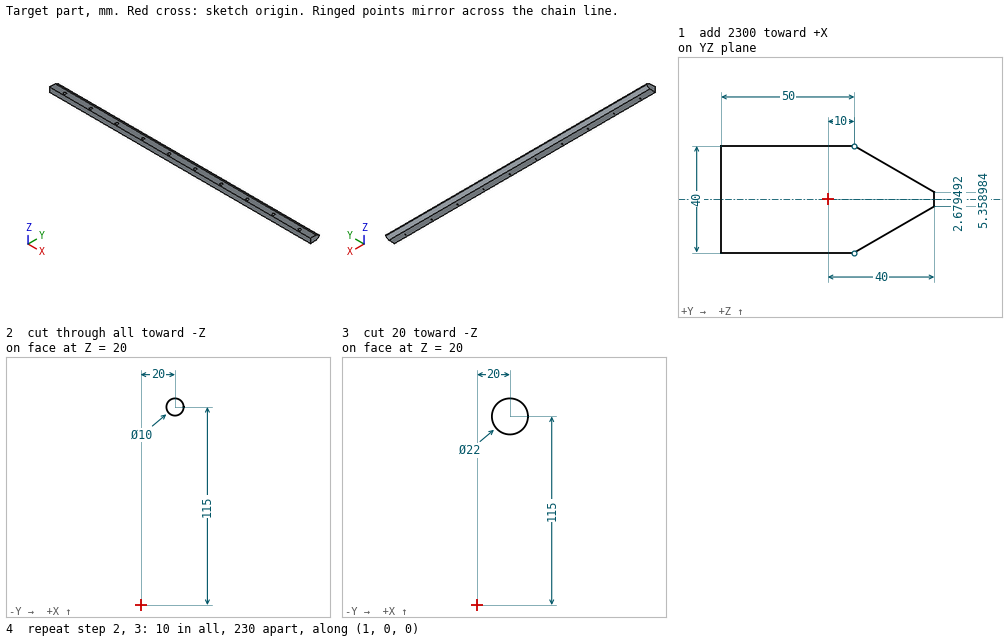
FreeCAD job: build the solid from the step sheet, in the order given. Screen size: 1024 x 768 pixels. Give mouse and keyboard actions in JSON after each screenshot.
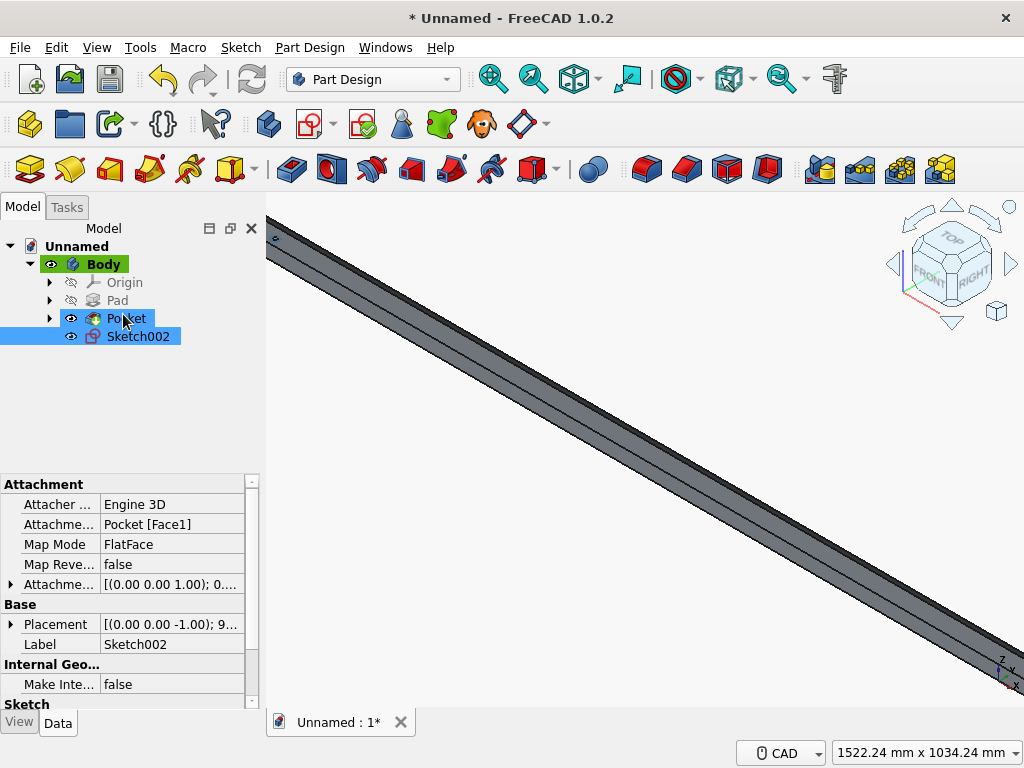
{"action": "left_click", "coordinate": [292, 170]}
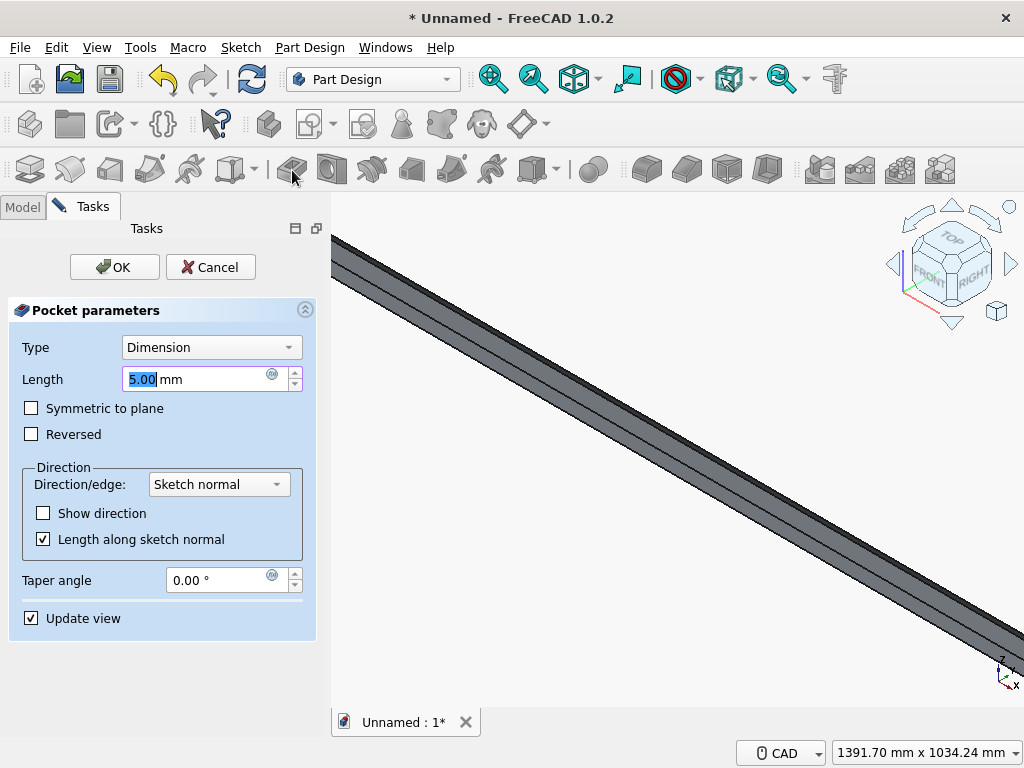
{"action": "type", "text": "20"}
{"action": "key", "text": "Tab"}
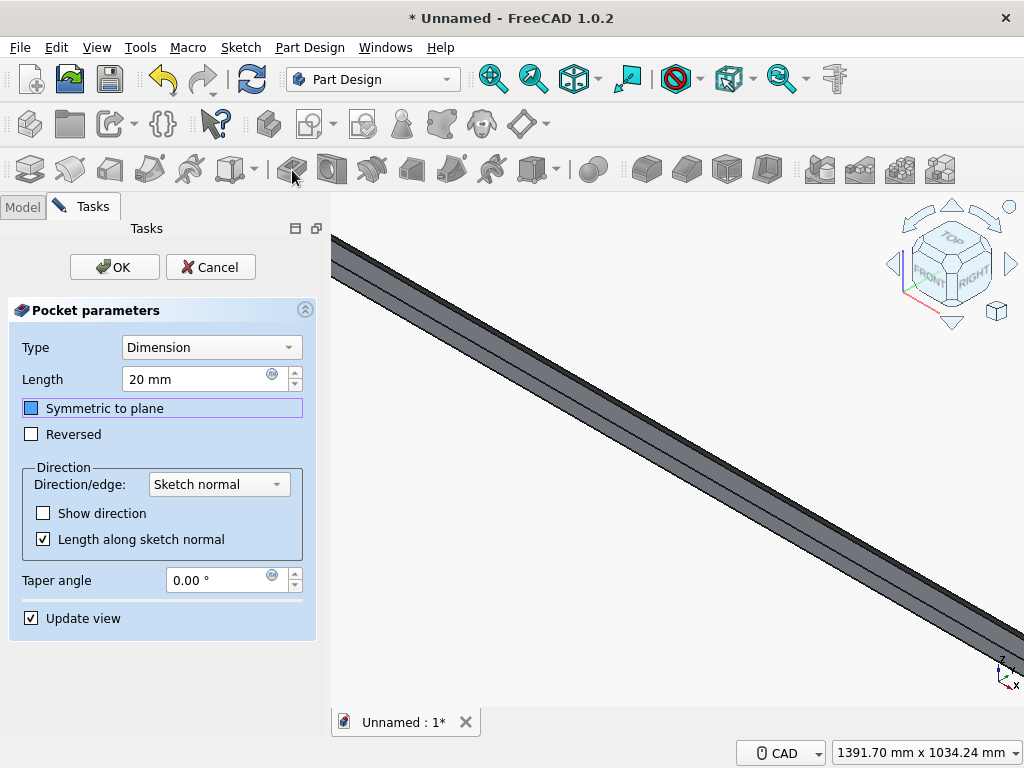
{"action": "left_click", "coordinate": [115, 267]}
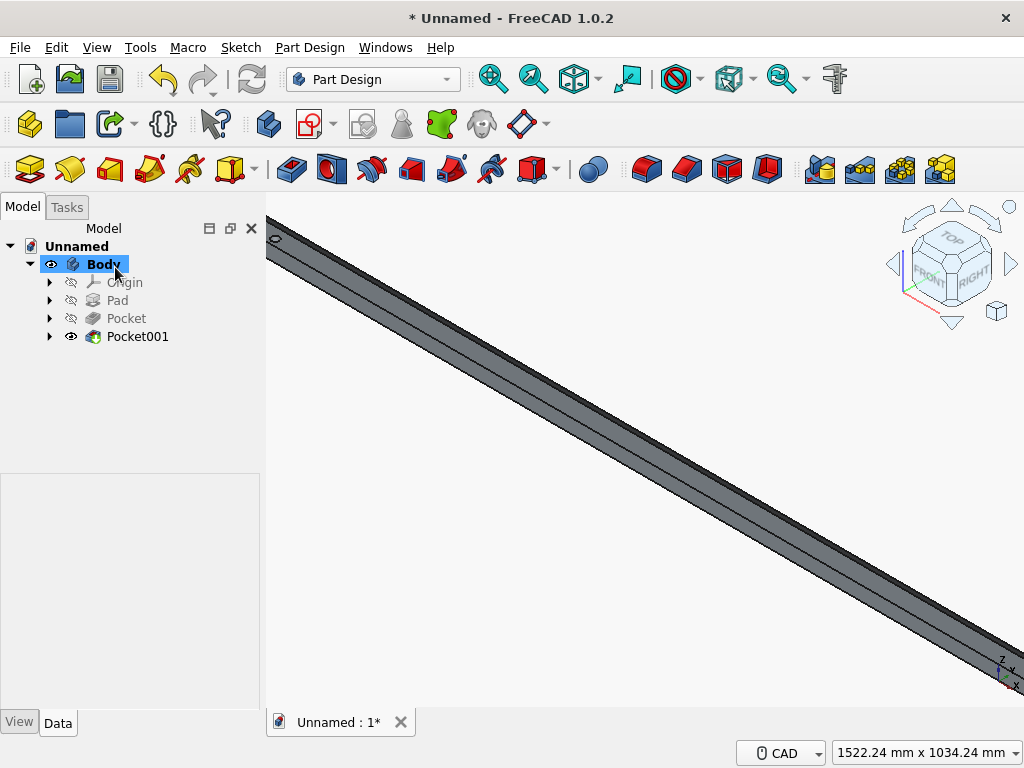
{"action": "key", "text": "v f"}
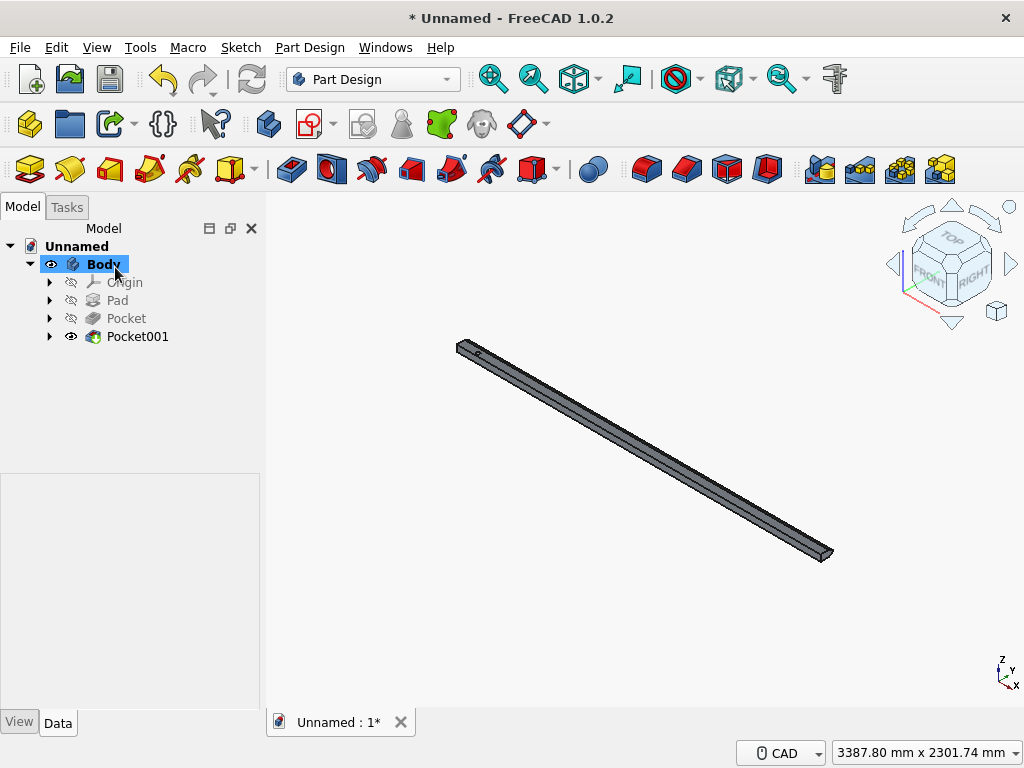
{"action": "left_click", "coordinate": [116, 318]}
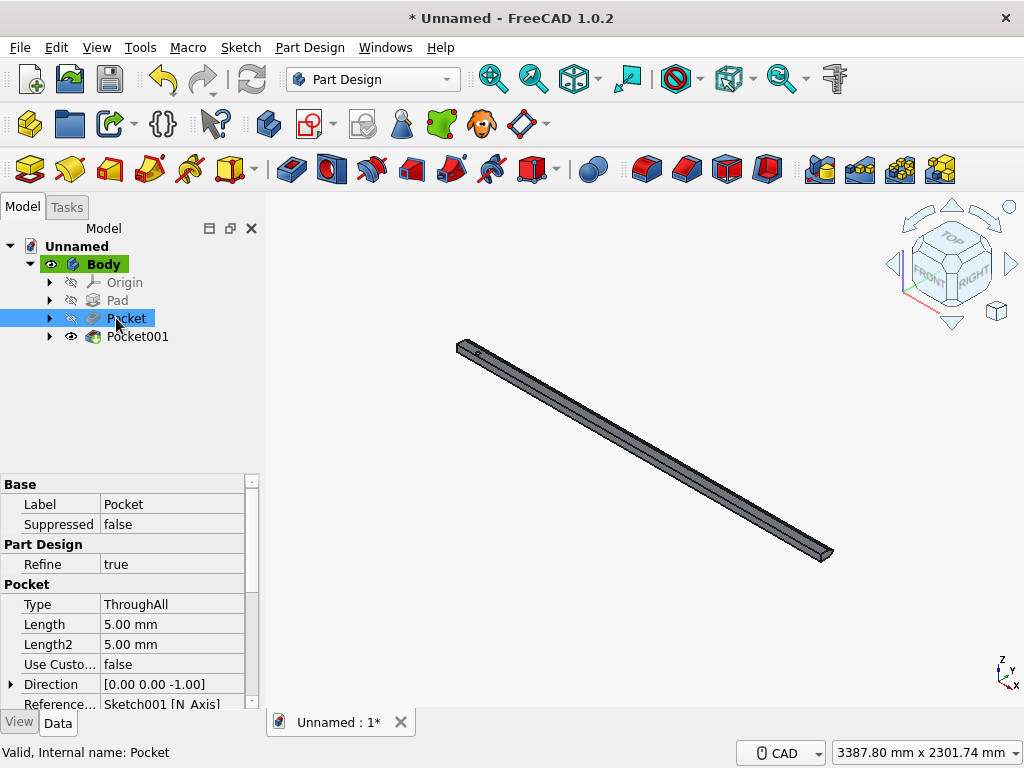
{"action": "left_click", "coordinate": [116, 336], "text": "ctrl"}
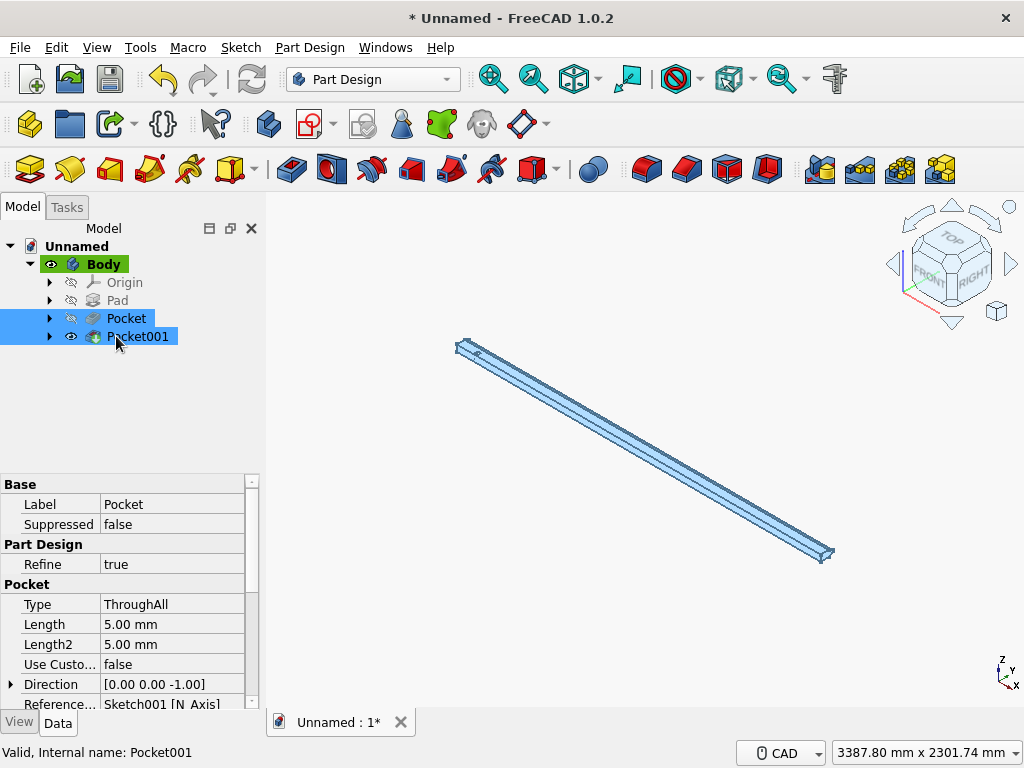
{"action": "left_click", "coordinate": [860, 170]}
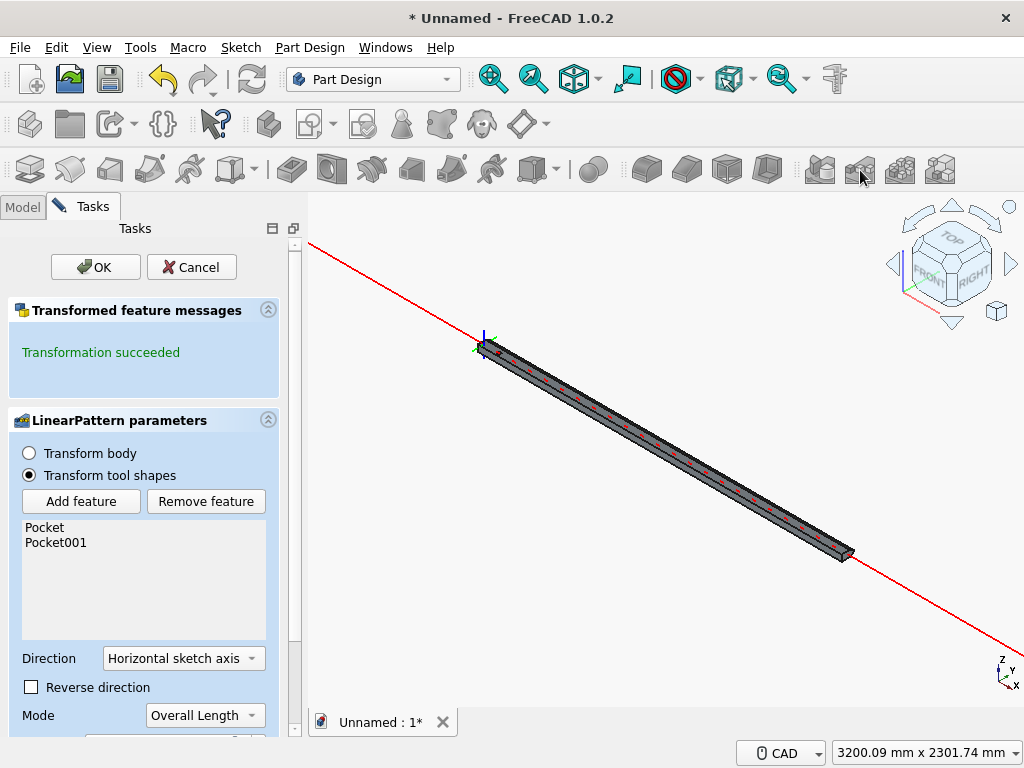
{"action": "left_click", "coordinate": [184, 658]}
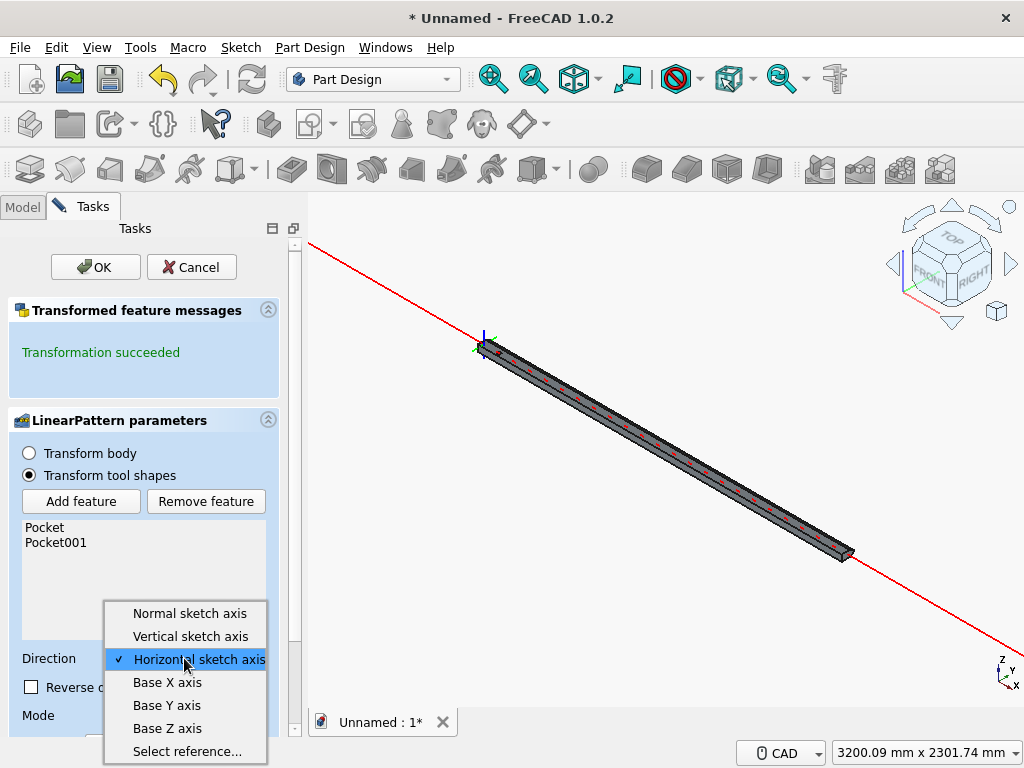
{"action": "left_click", "coordinate": [184, 682]}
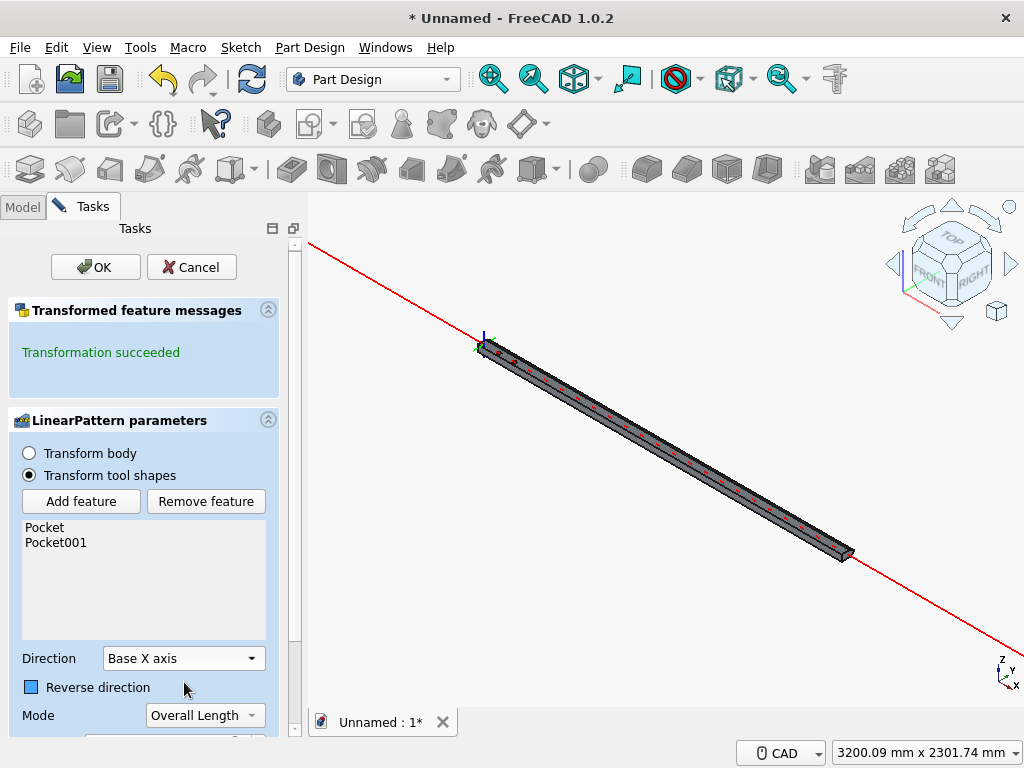
{"action": "left_click", "coordinate": [206, 716]}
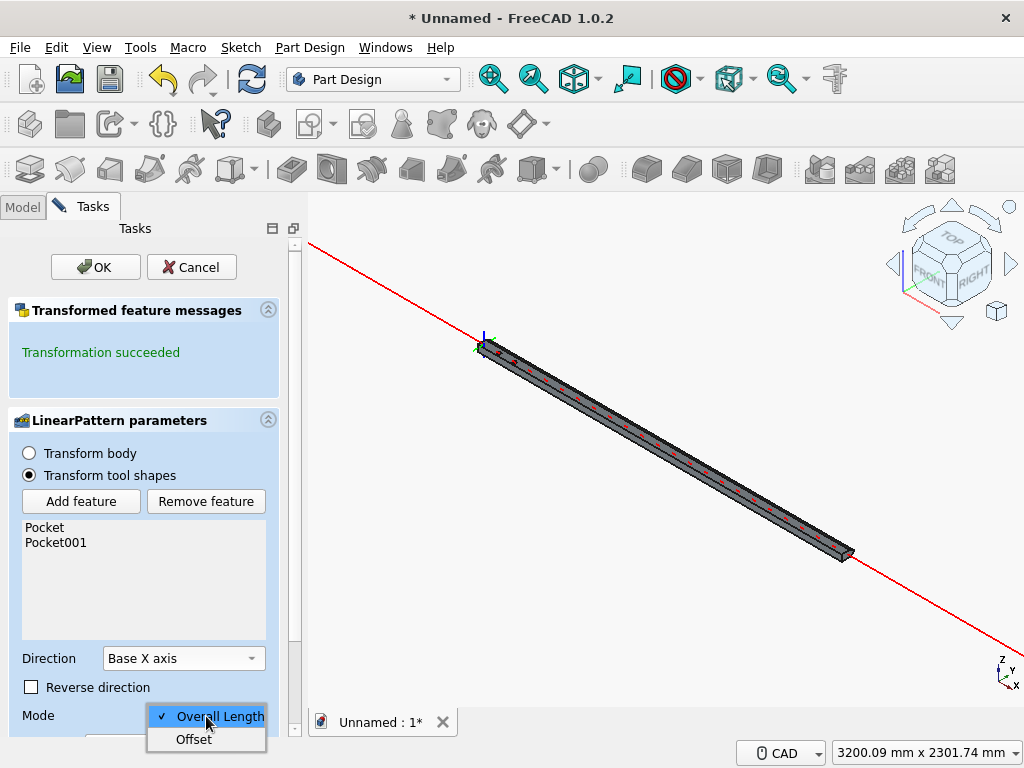
{"action": "left_click", "coordinate": [206, 740]}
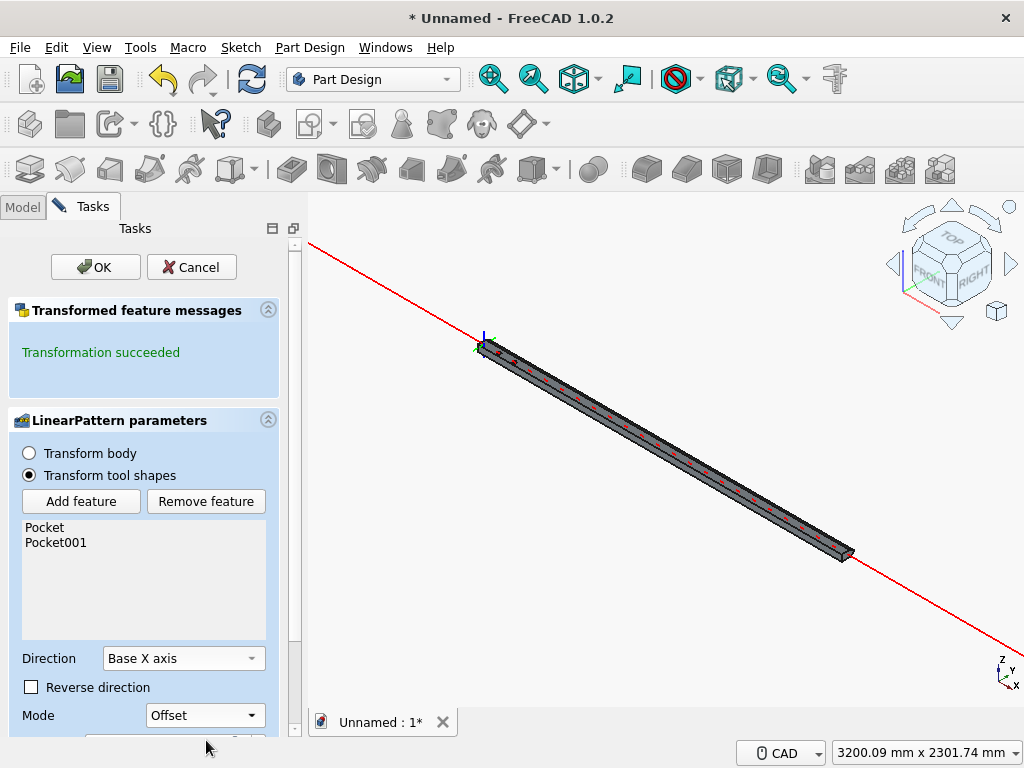
{"action": "scroll", "coordinate": [295, 487], "scroll_direction": "down", "scroll_amount": 2}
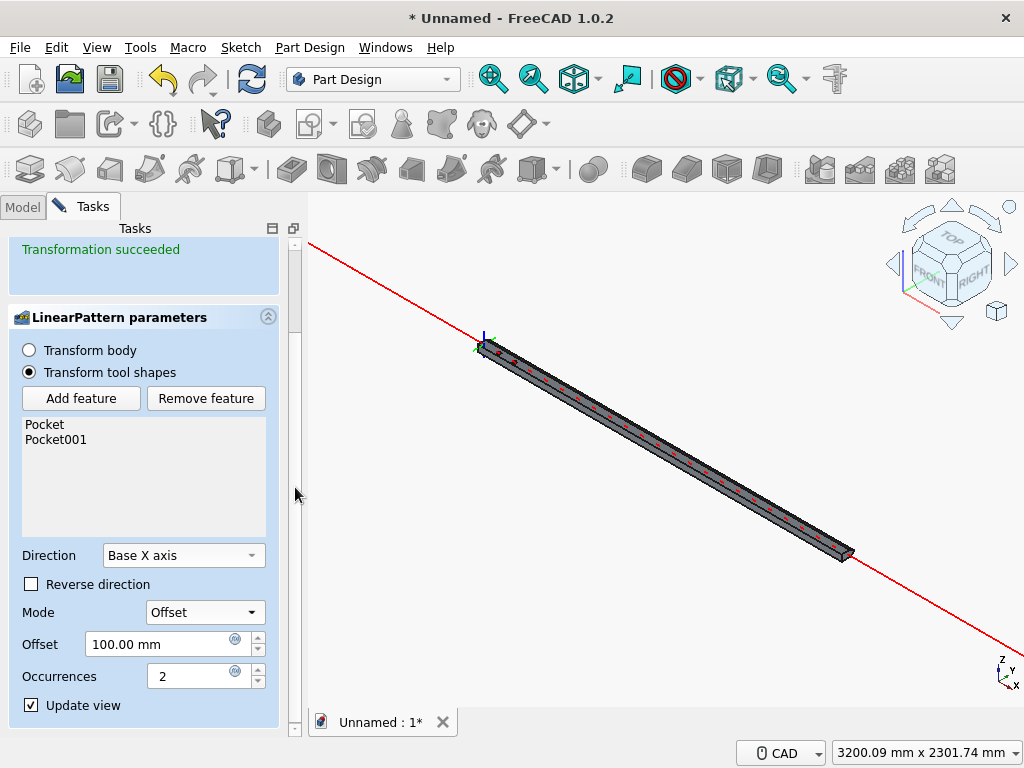
{"action": "triple_click", "coordinate": [168, 644]}